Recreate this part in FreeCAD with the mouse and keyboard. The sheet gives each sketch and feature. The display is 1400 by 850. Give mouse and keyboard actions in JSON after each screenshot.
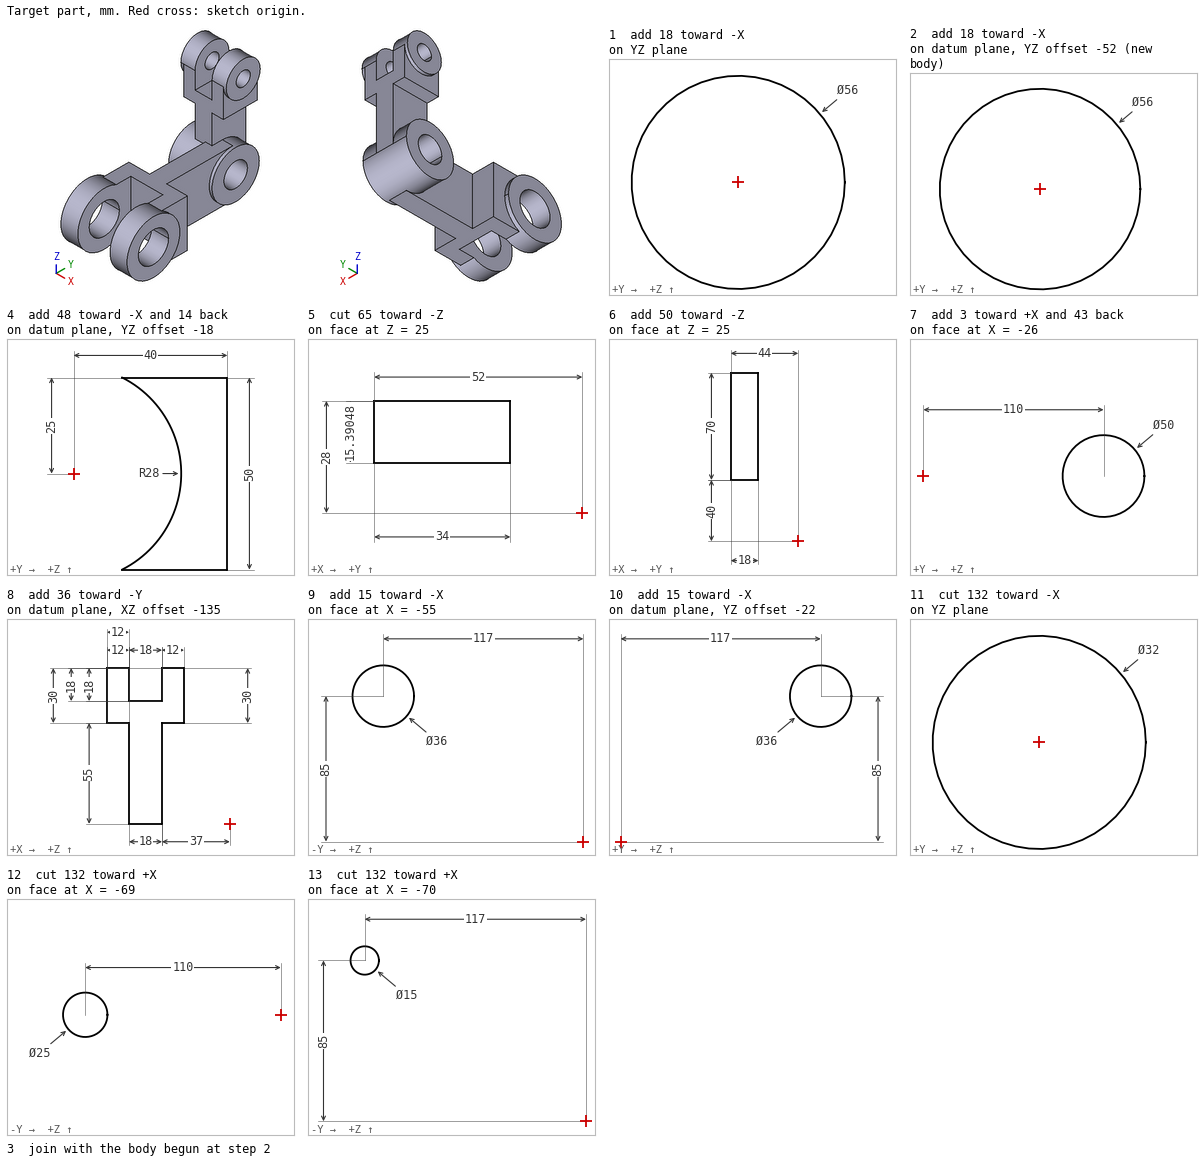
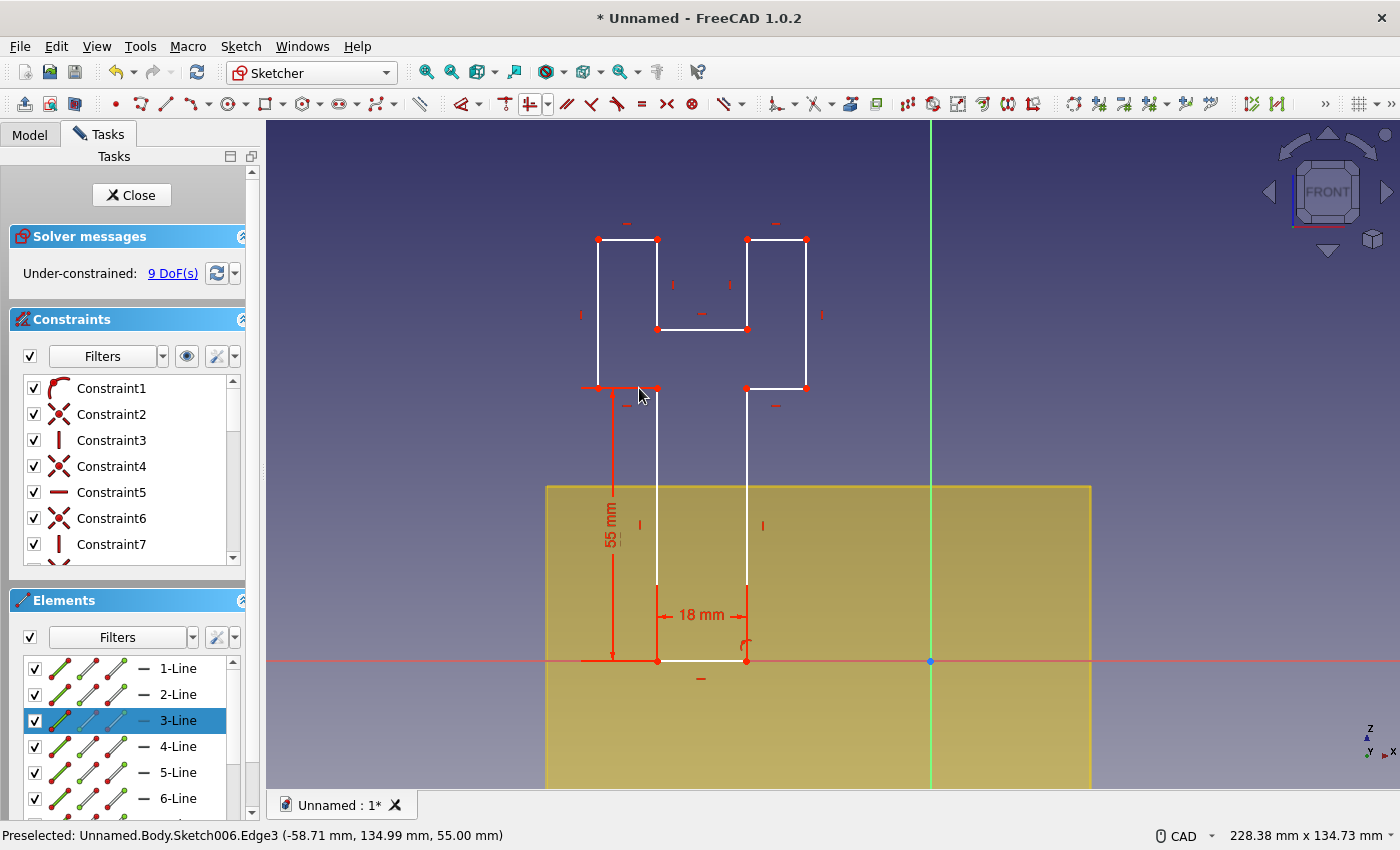
{"action": "key", "text": "l"}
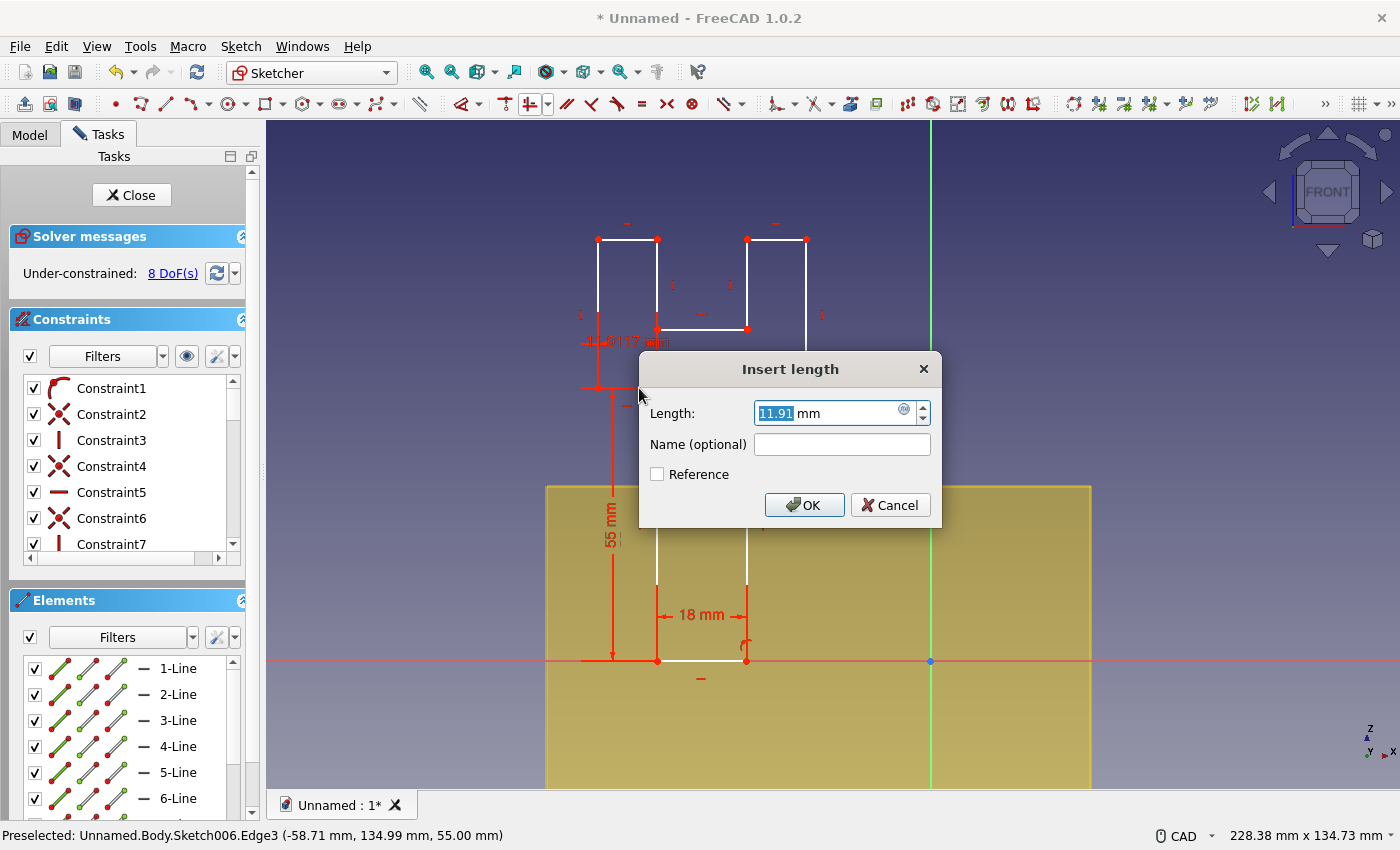
{"action": "type", "text": "12"}
{"action": "key", "text": "Return"}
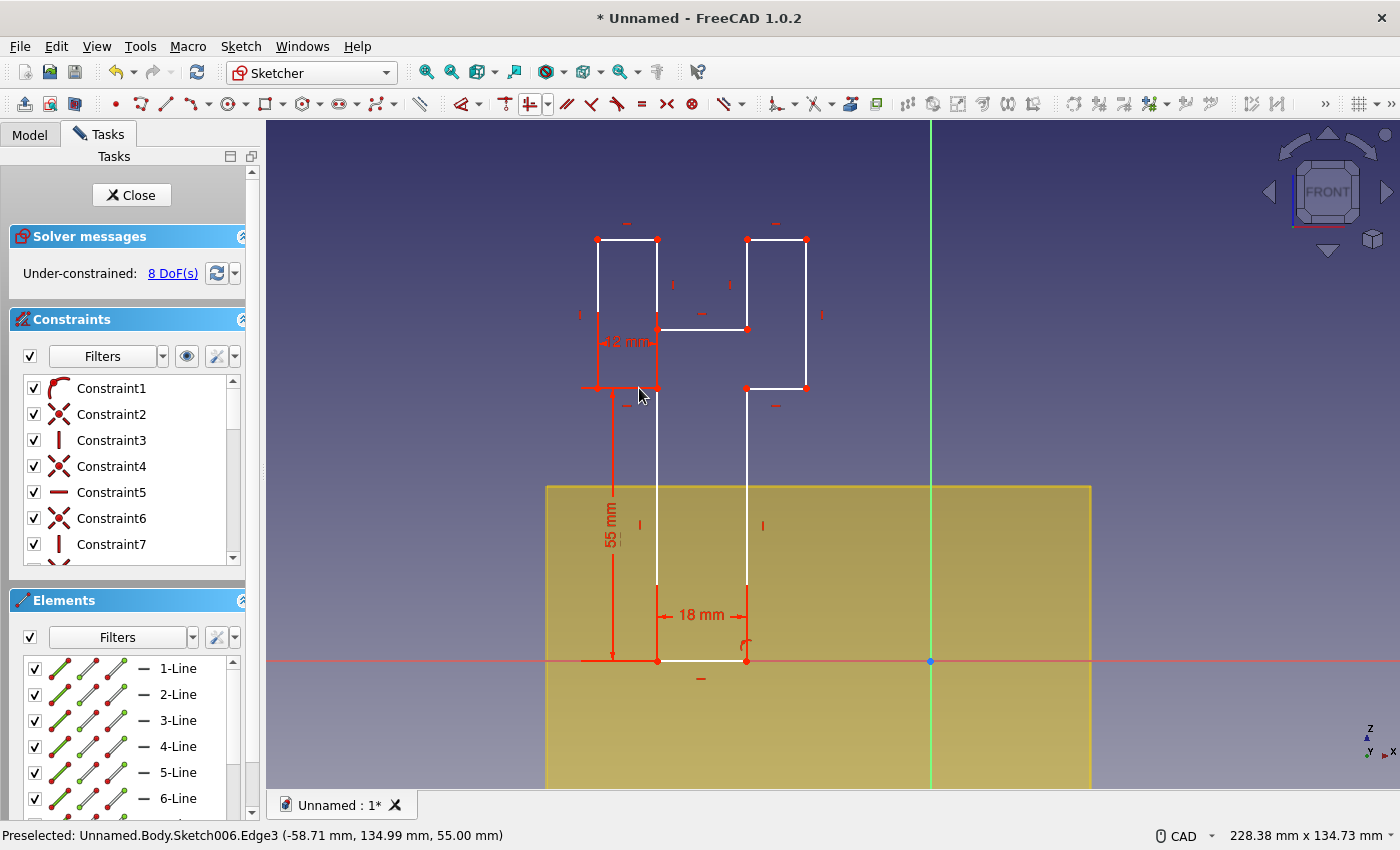
{"action": "left_click", "coordinate": [598, 344]}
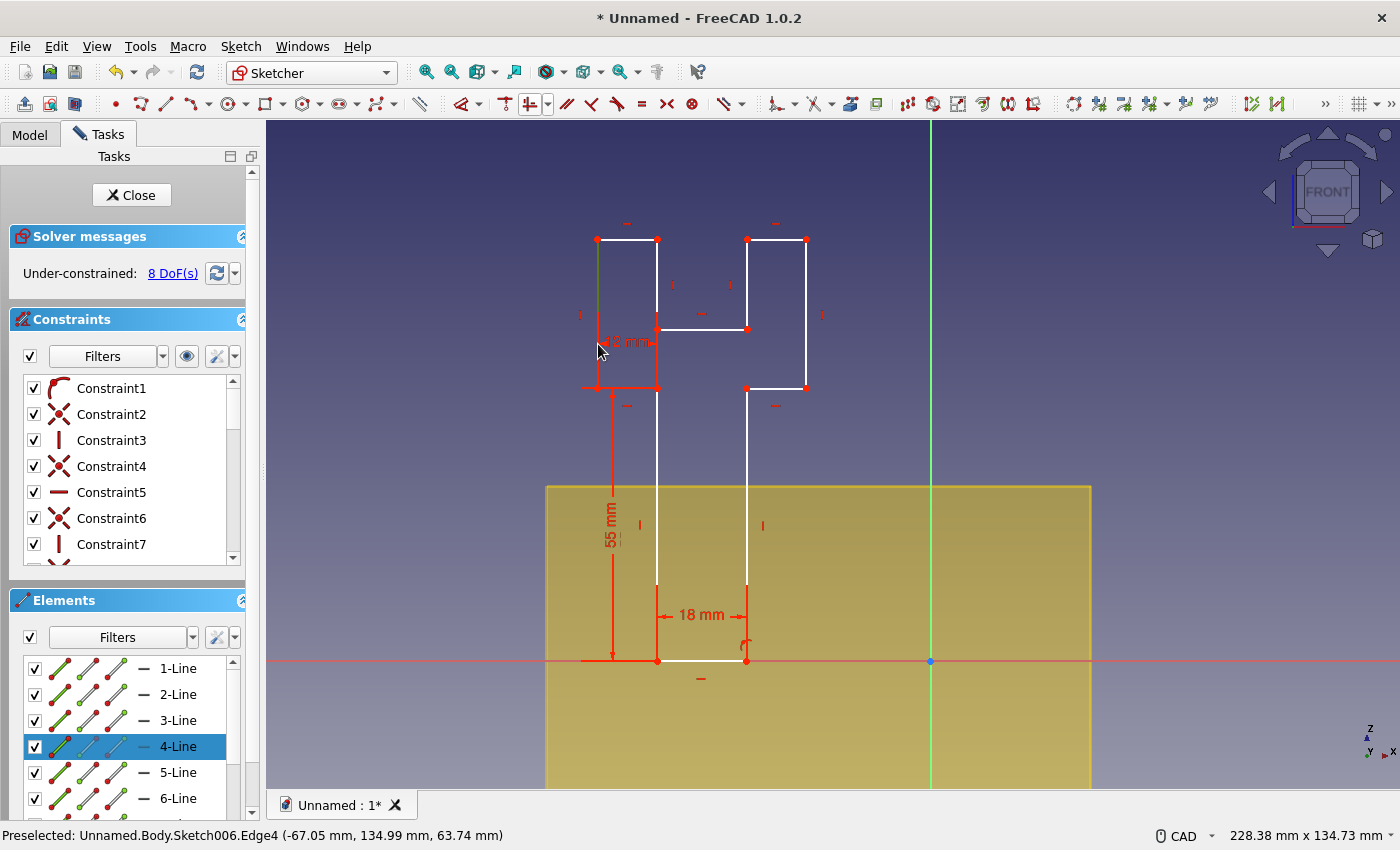
{"action": "key", "text": "i"}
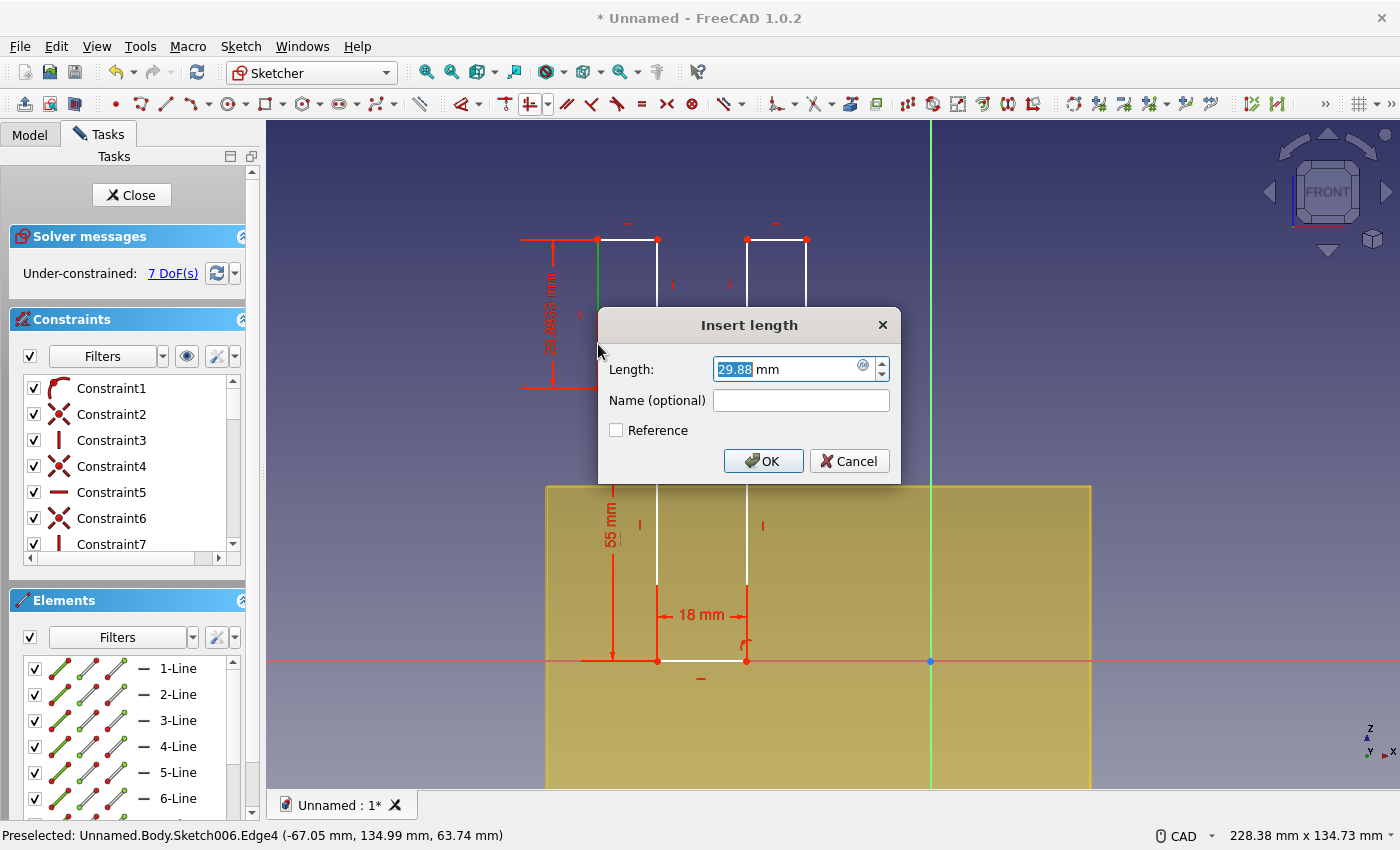
{"action": "type", "text": "30"}
{"action": "key", "text": "Return"}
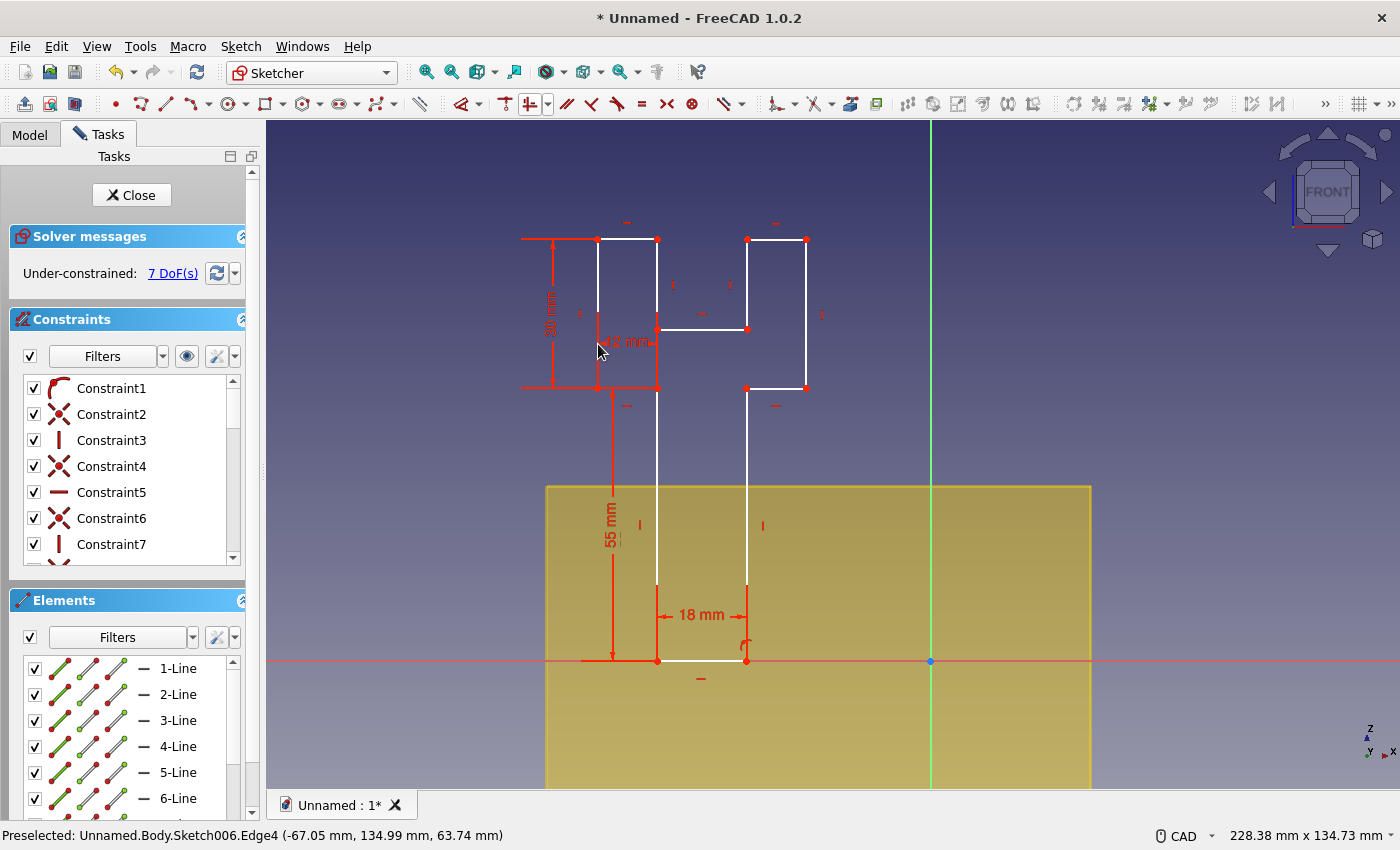
{"action": "left_click", "coordinate": [615, 239]}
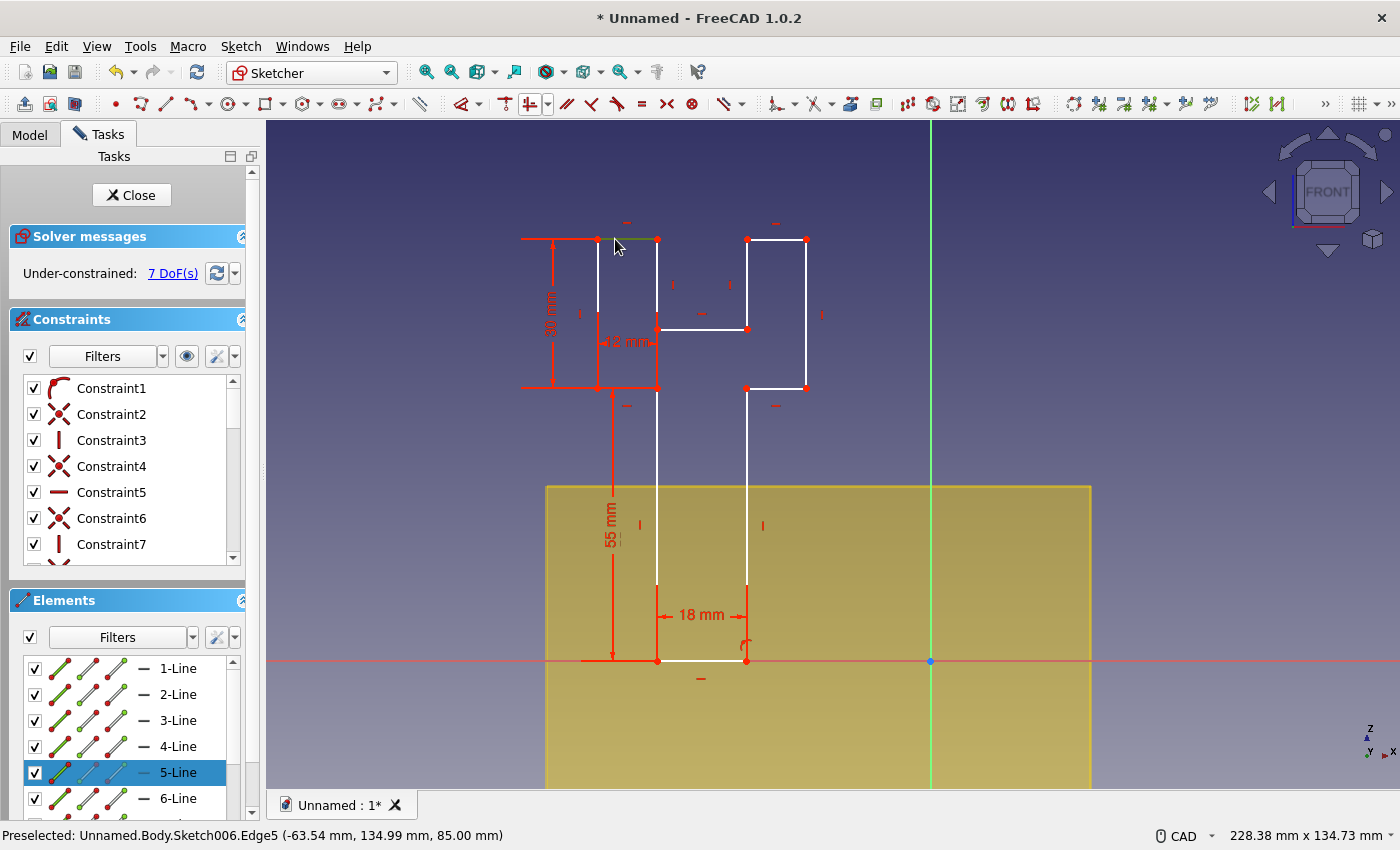
{"action": "key", "text": "l"}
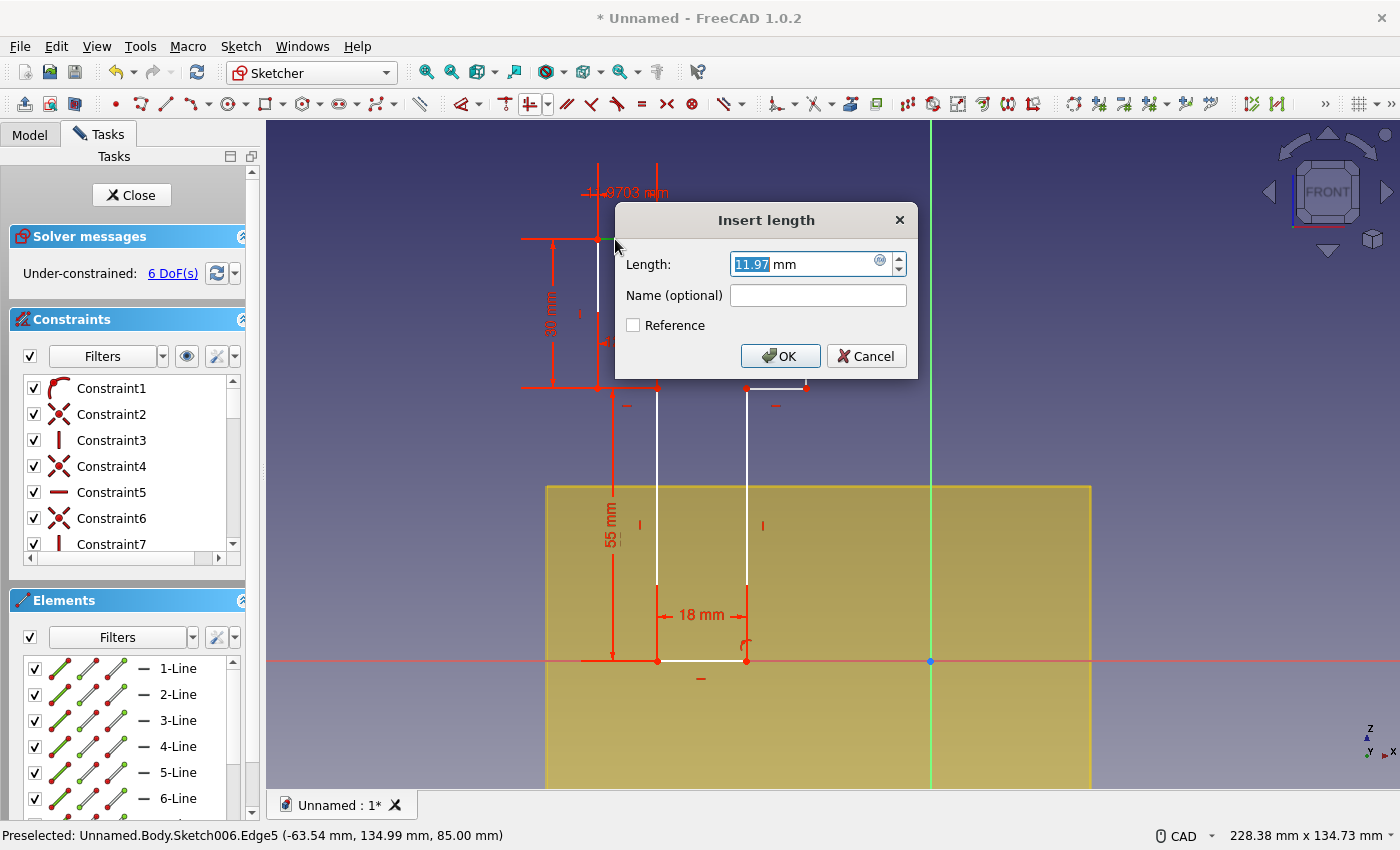
{"action": "type", "text": "12"}
{"action": "key", "text": "Return"}